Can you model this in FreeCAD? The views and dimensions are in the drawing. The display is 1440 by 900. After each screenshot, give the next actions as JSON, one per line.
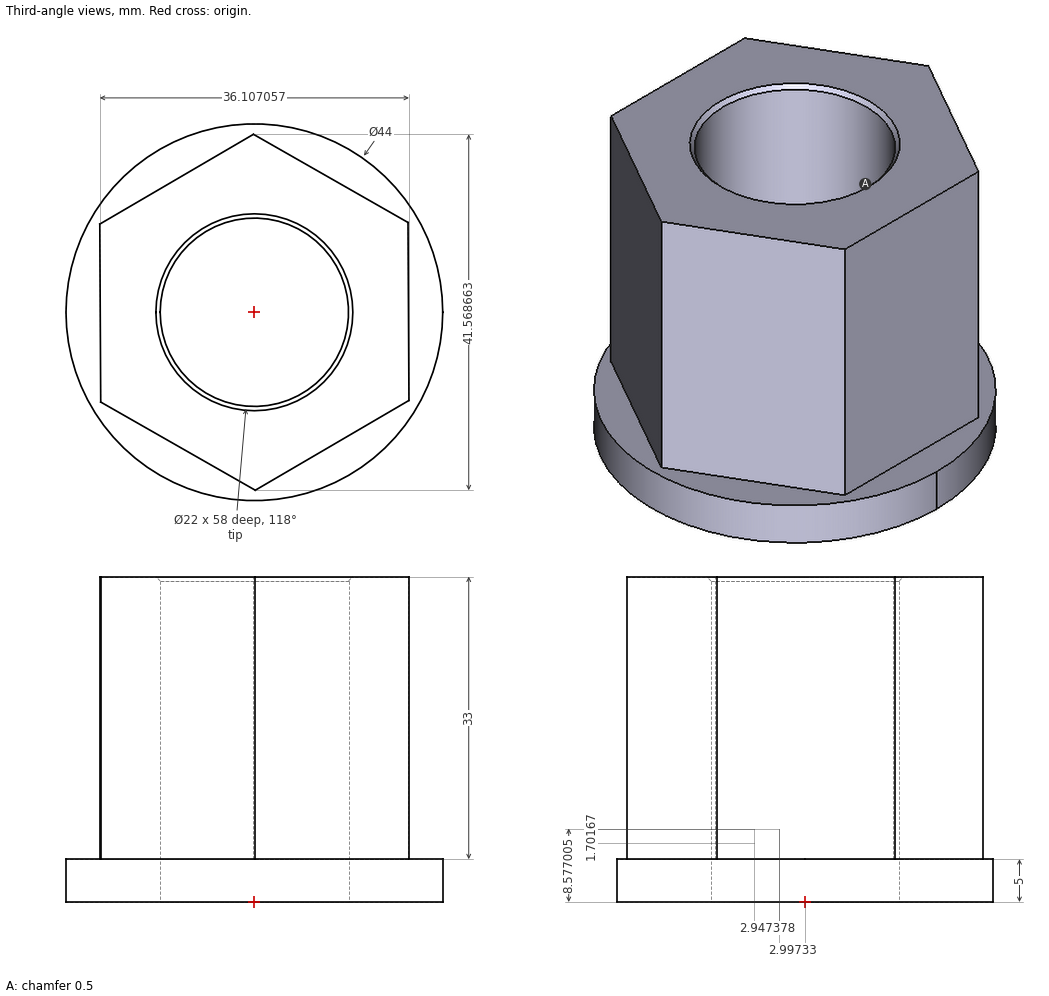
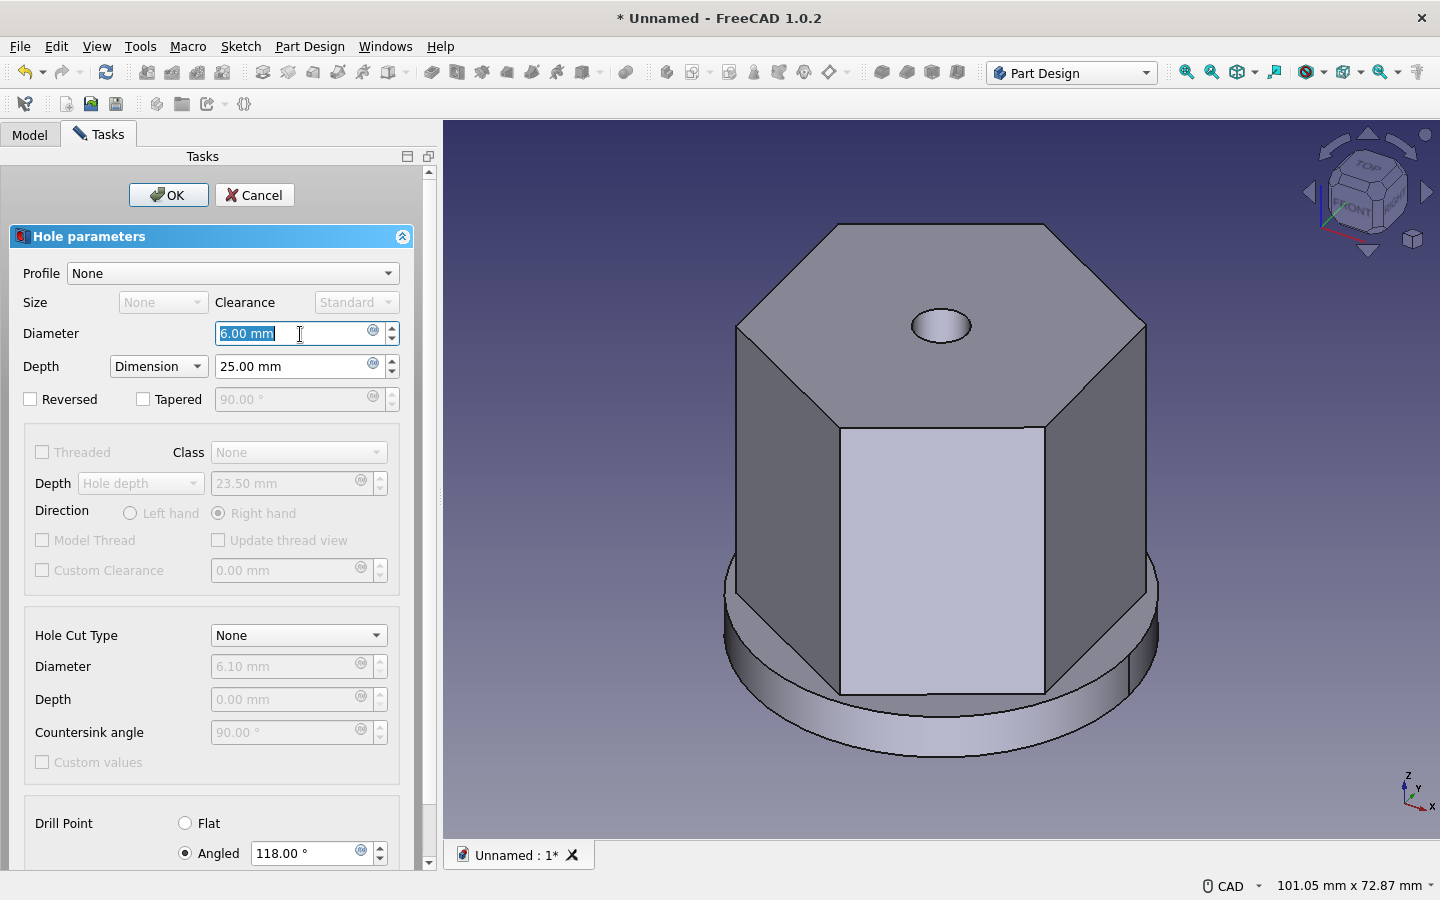
{"action": "type", "text": "22"}
{"action": "key", "text": "Tab"}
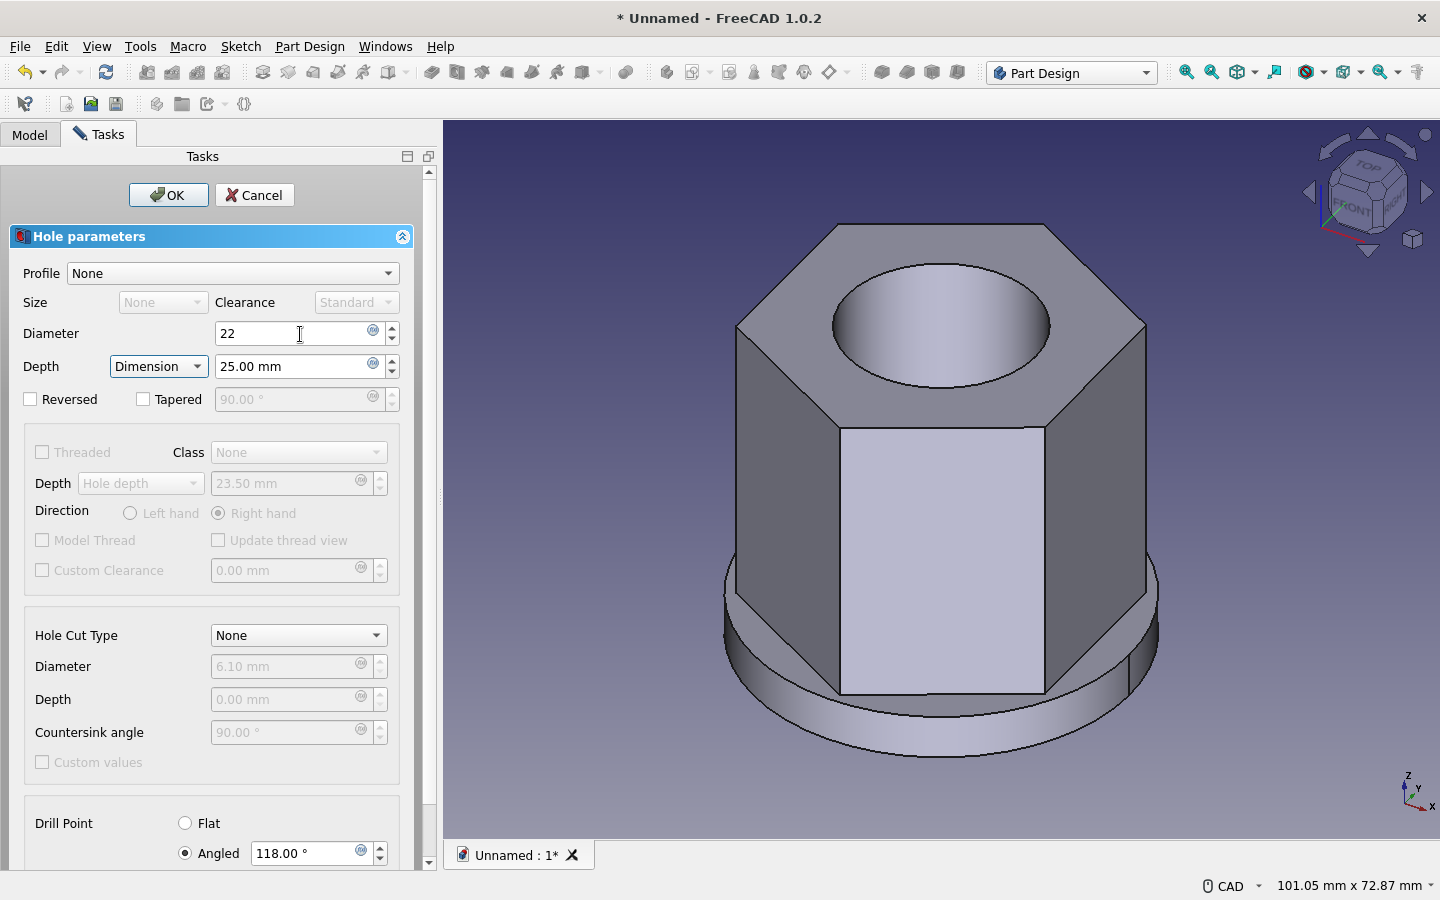
{"action": "triple_click", "coordinate": [300, 366]}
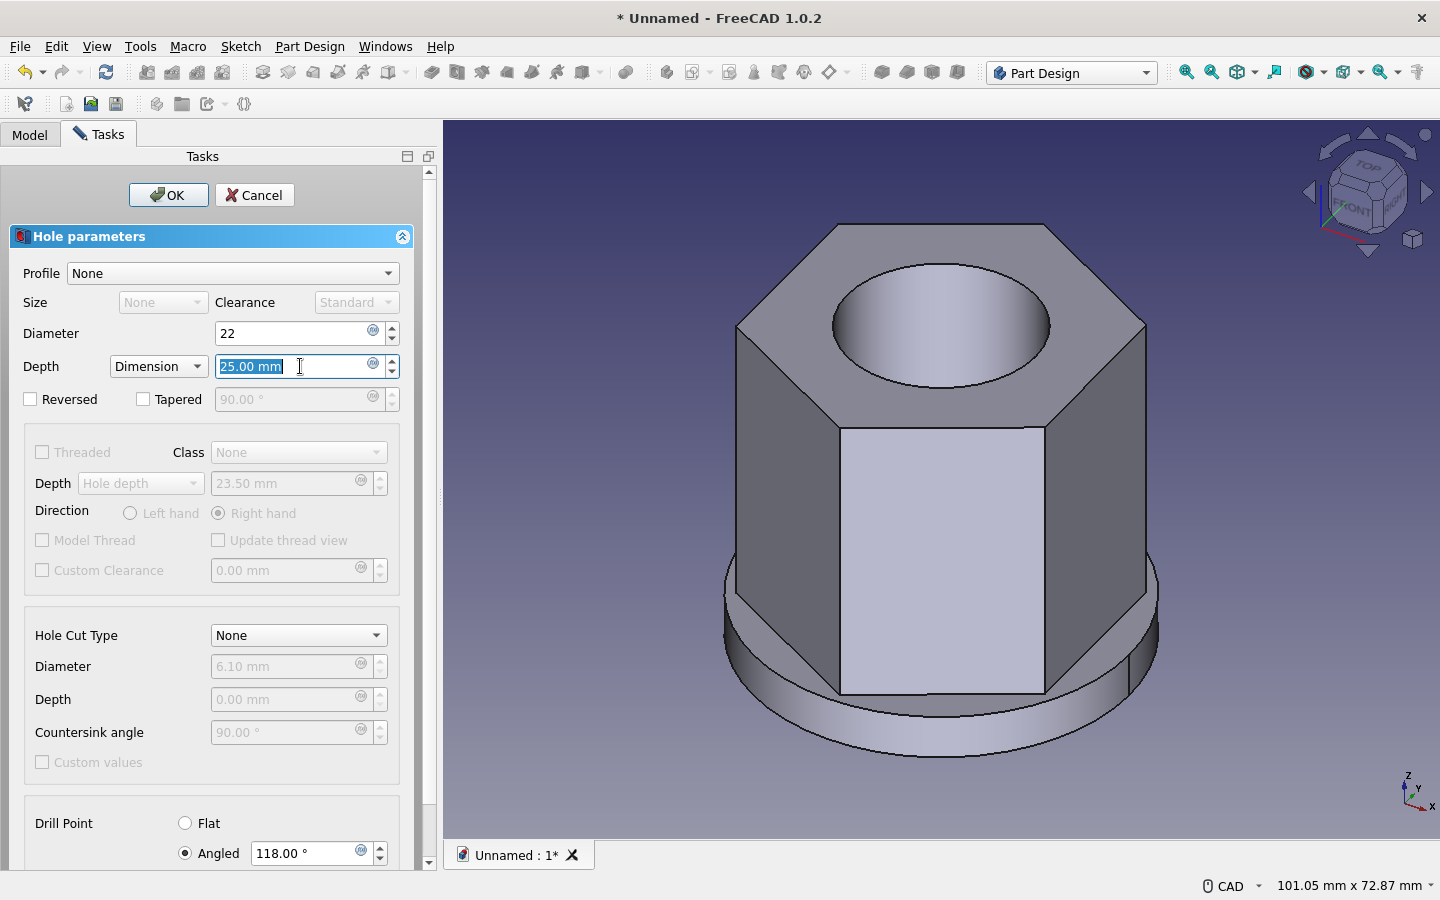
{"action": "type", "text": "58"}
{"action": "key", "text": "Tab"}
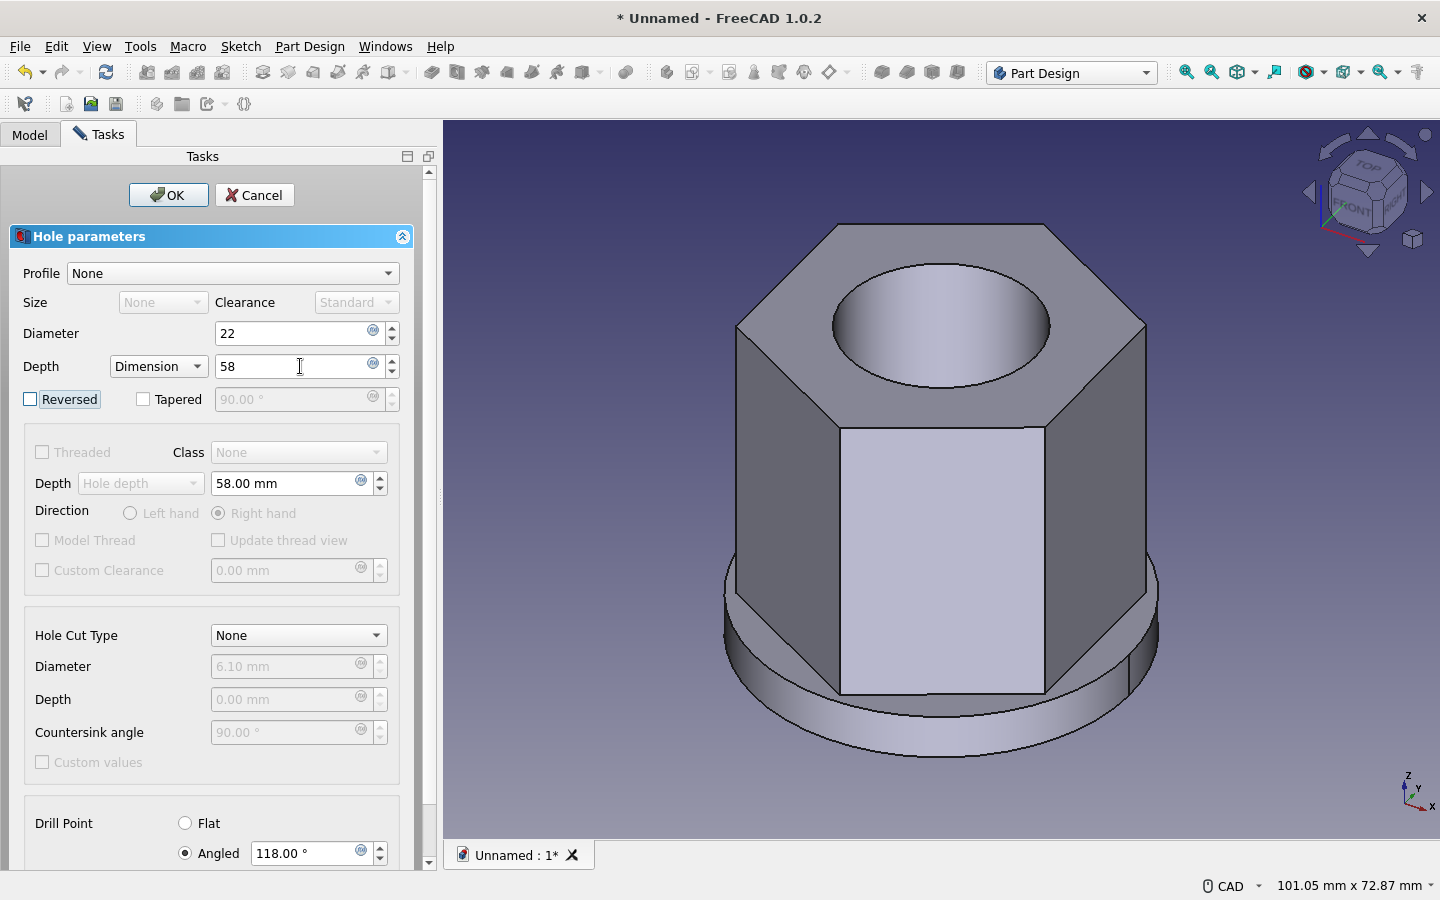
{"action": "left_click", "coordinate": [169, 195]}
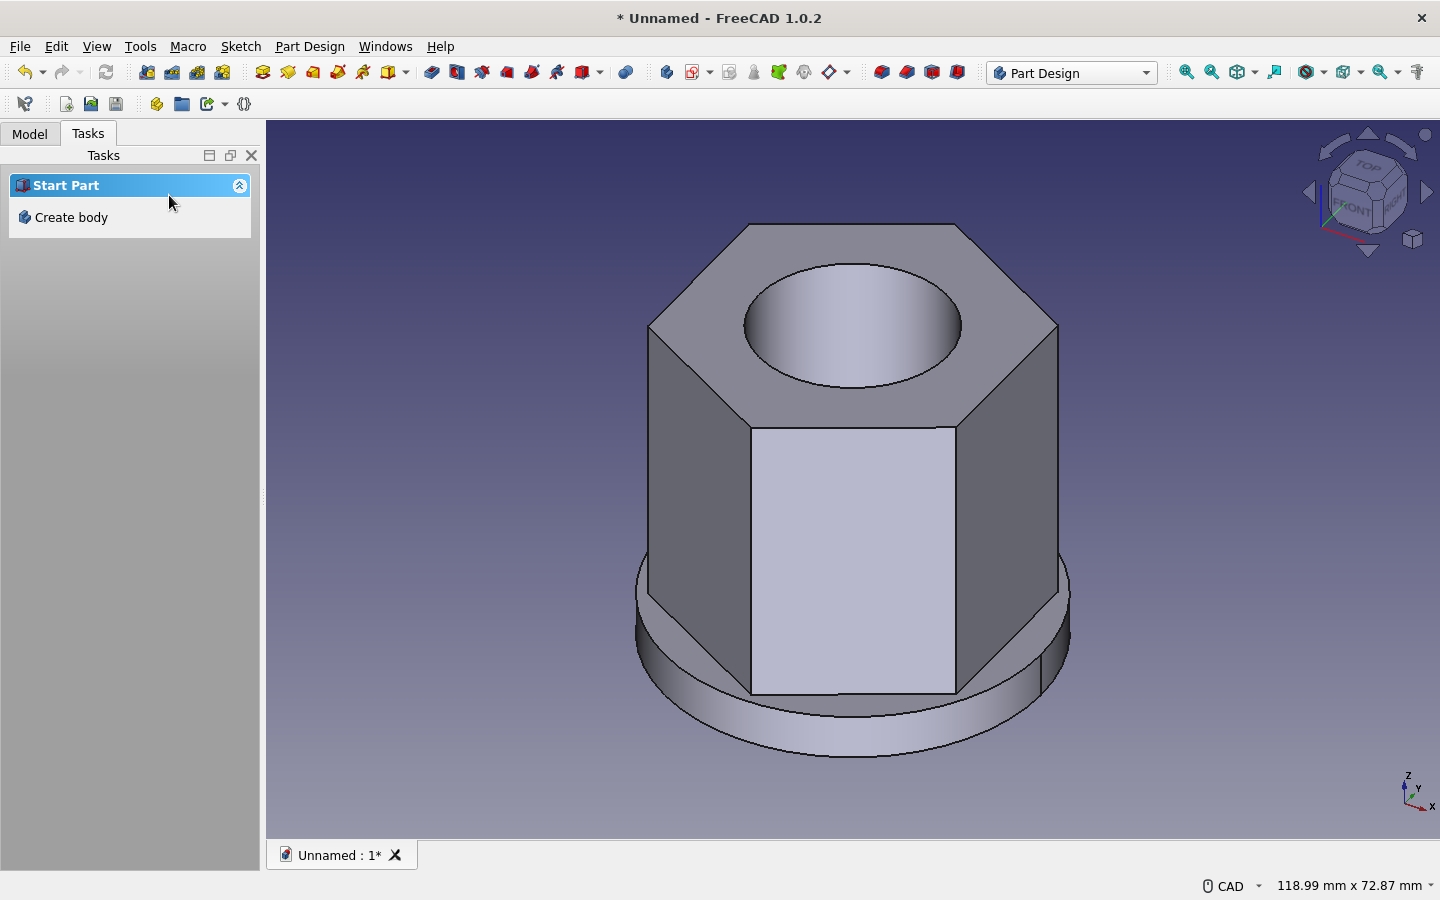
{"action": "left_click", "coordinate": [759, 294]}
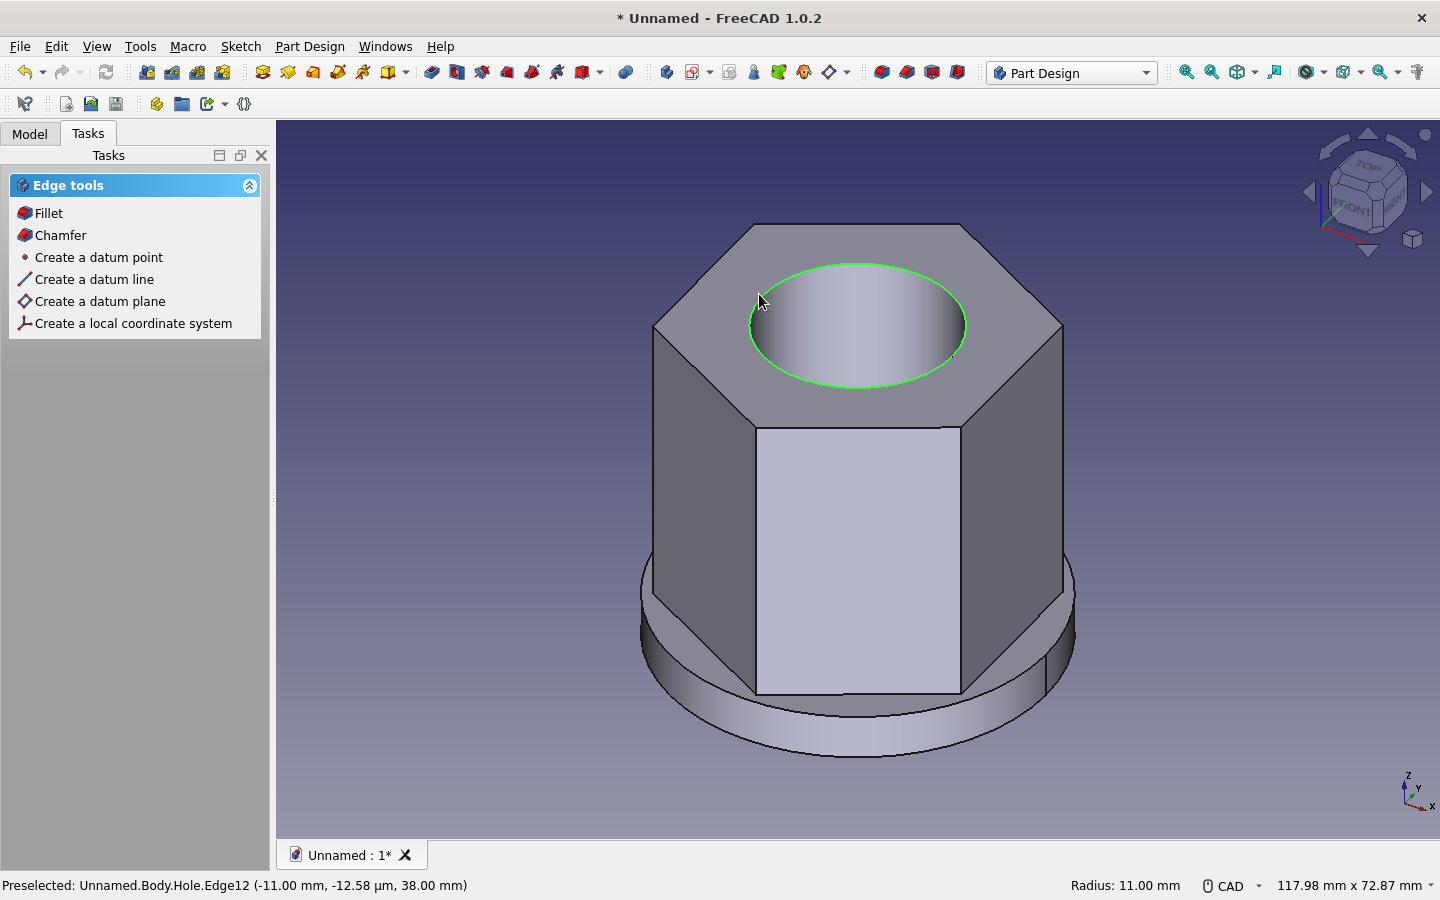
{"action": "left_click", "coordinate": [907, 72]}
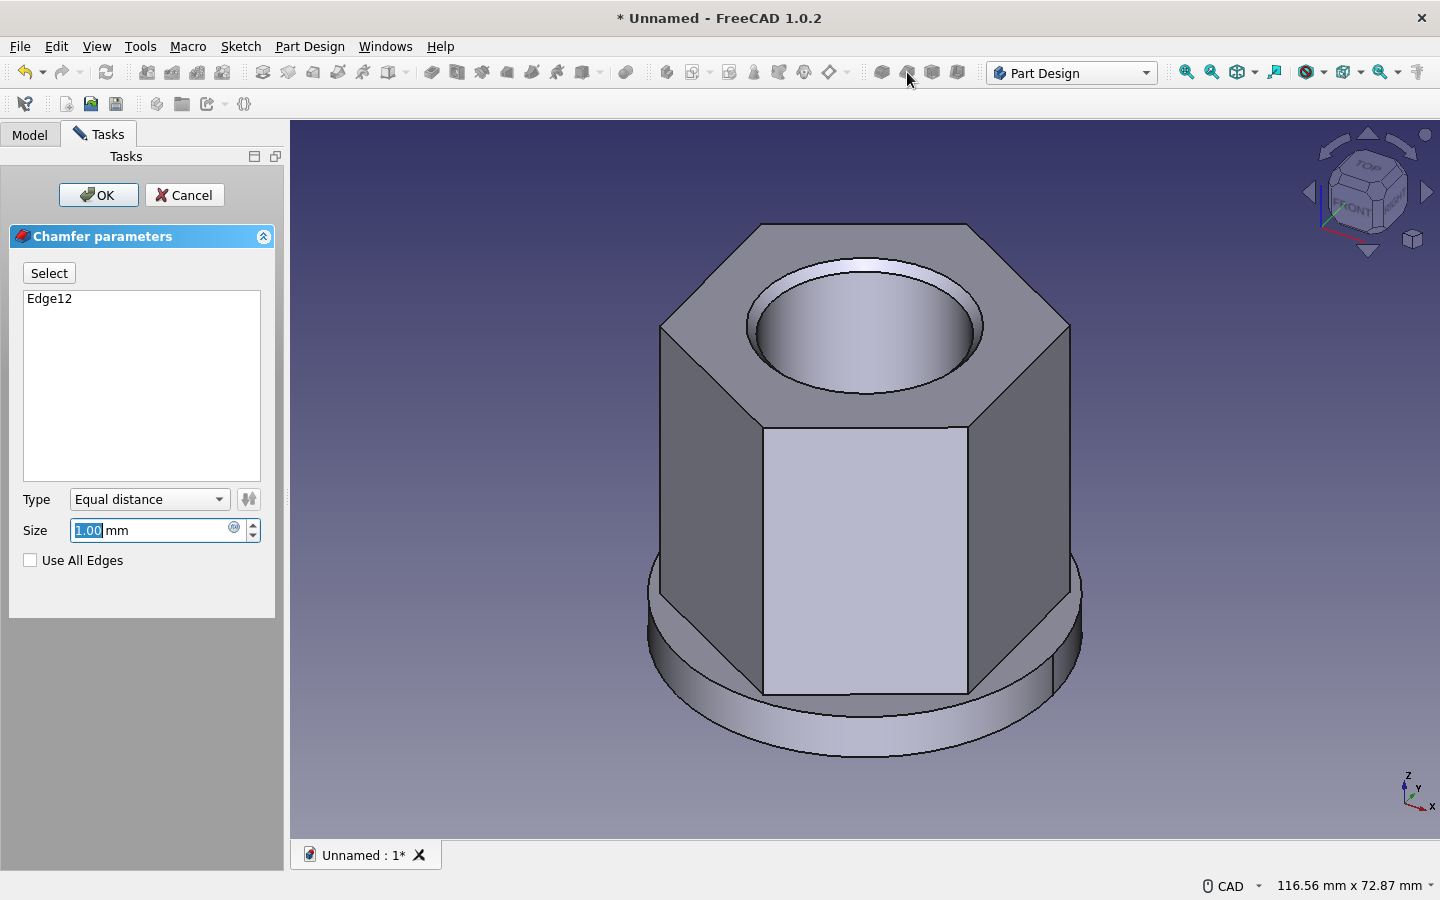
{"action": "type", "text": "0.5"}
{"action": "key", "text": "Tab"}